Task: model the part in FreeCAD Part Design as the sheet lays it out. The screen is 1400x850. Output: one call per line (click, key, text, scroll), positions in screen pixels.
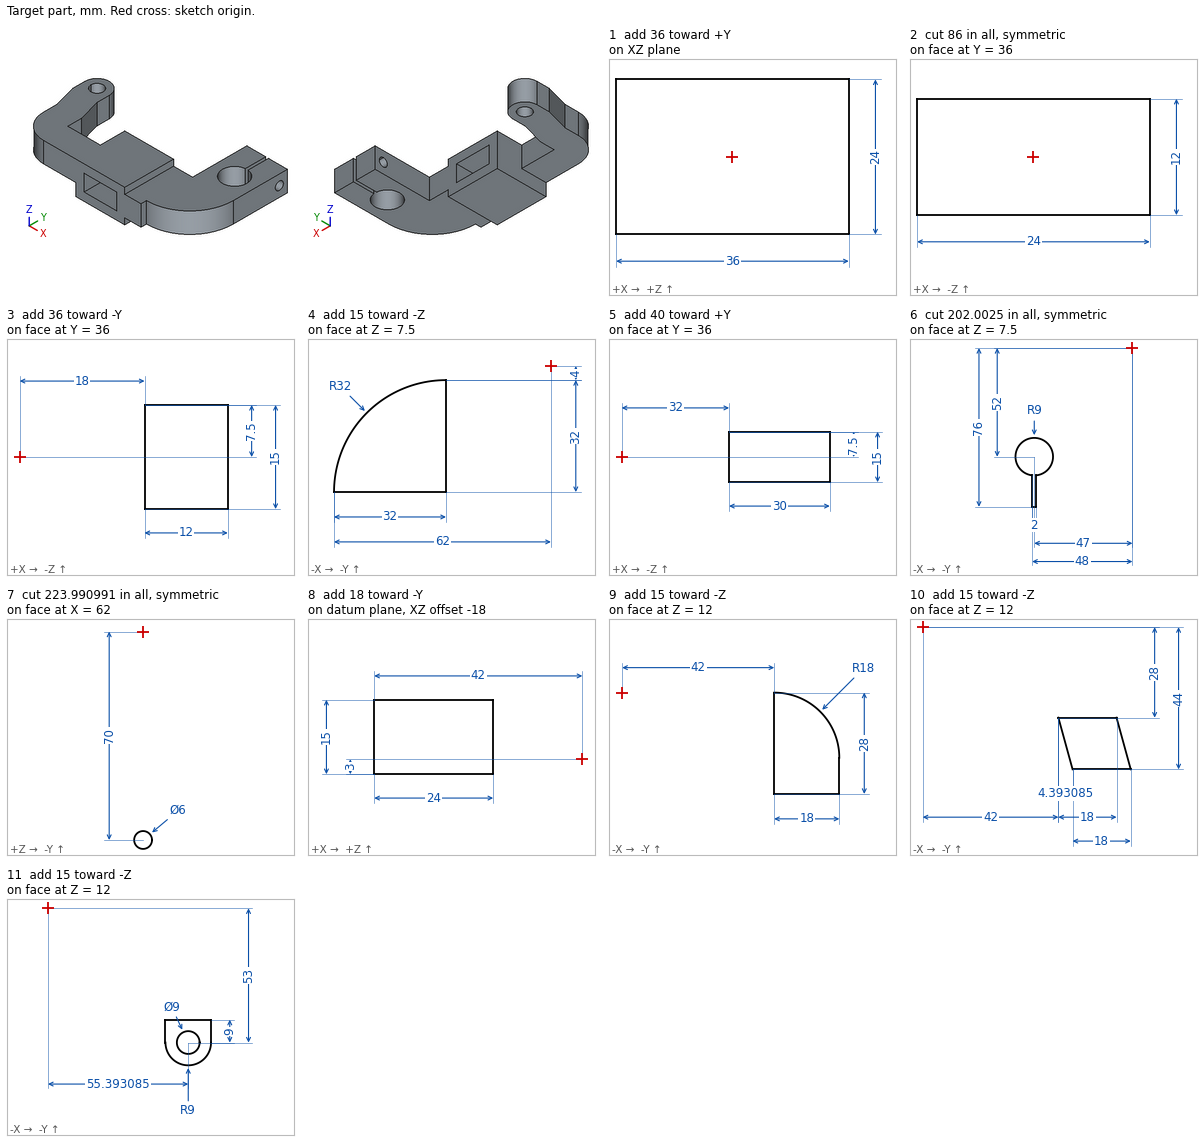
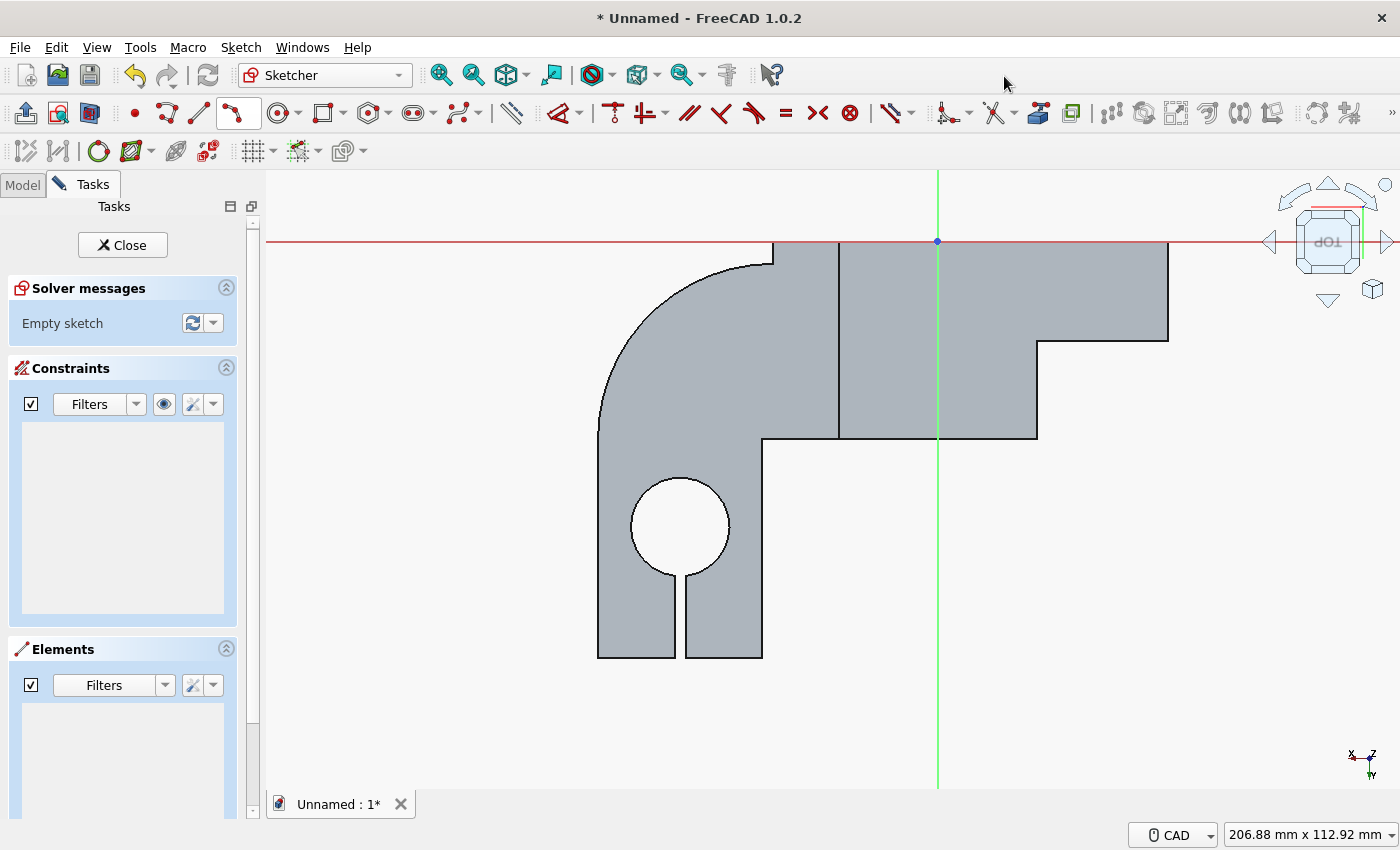
scroll(764, 480, down, 5)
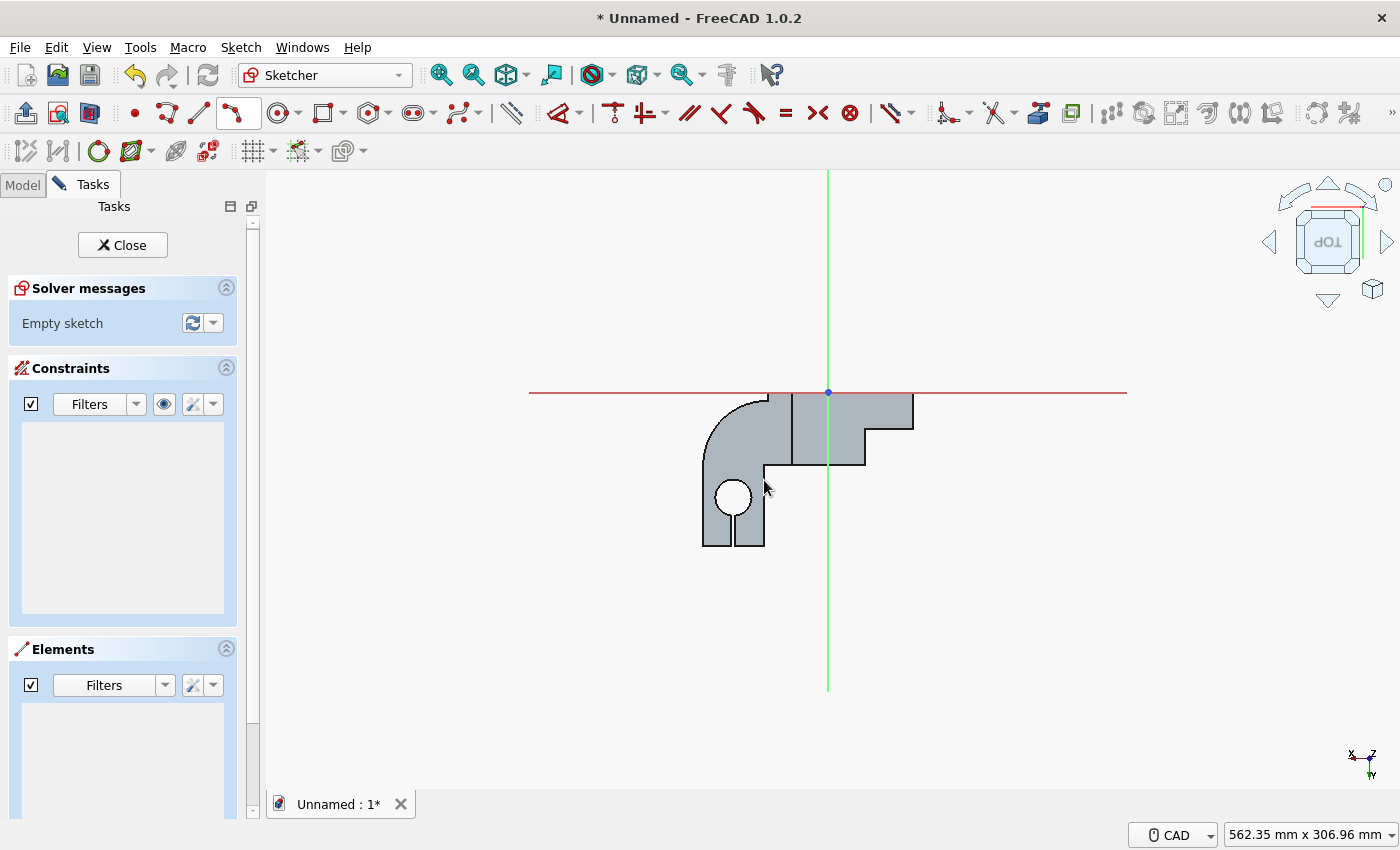
scroll(913, 409, up, 9)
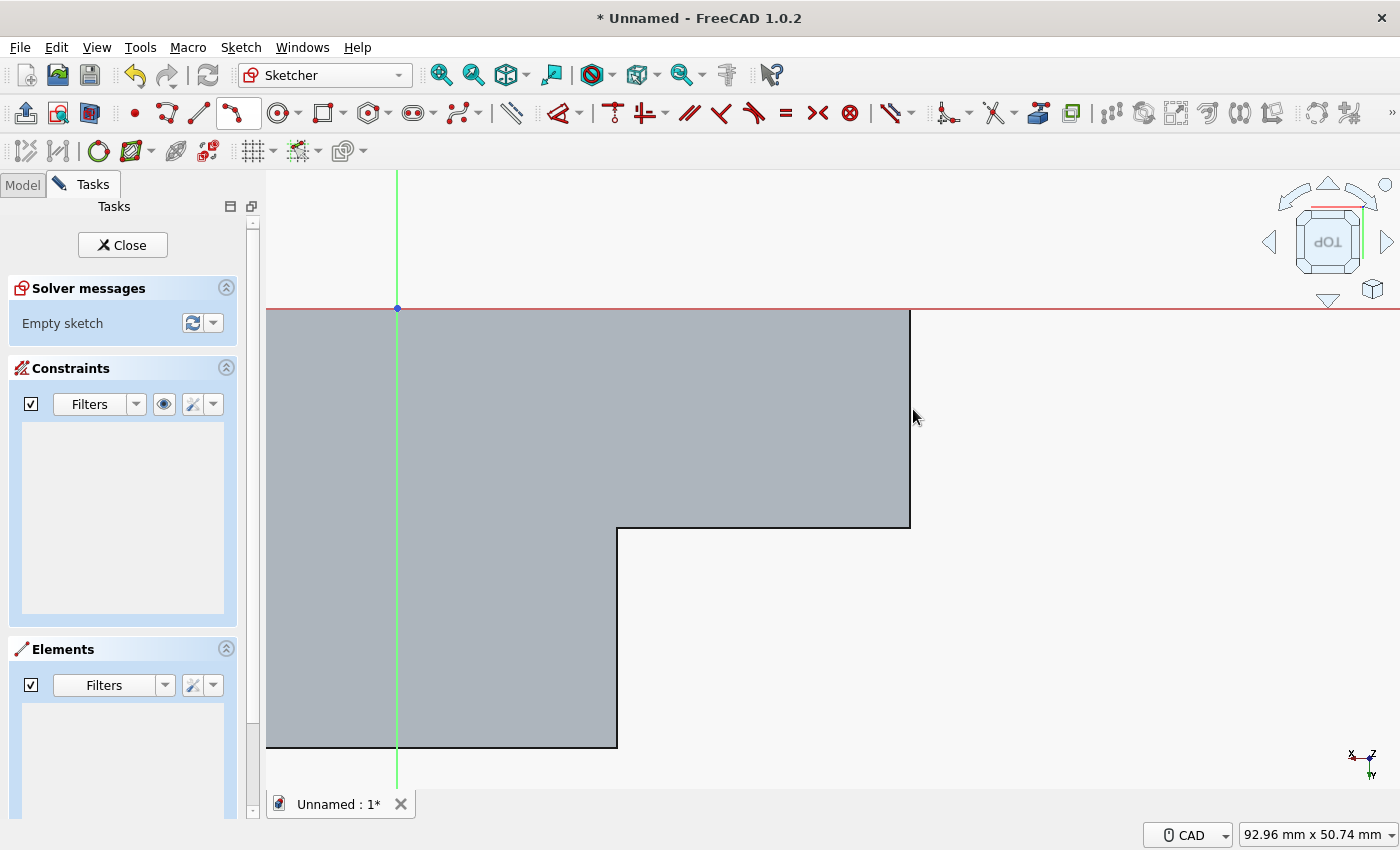
key(g)
key(m)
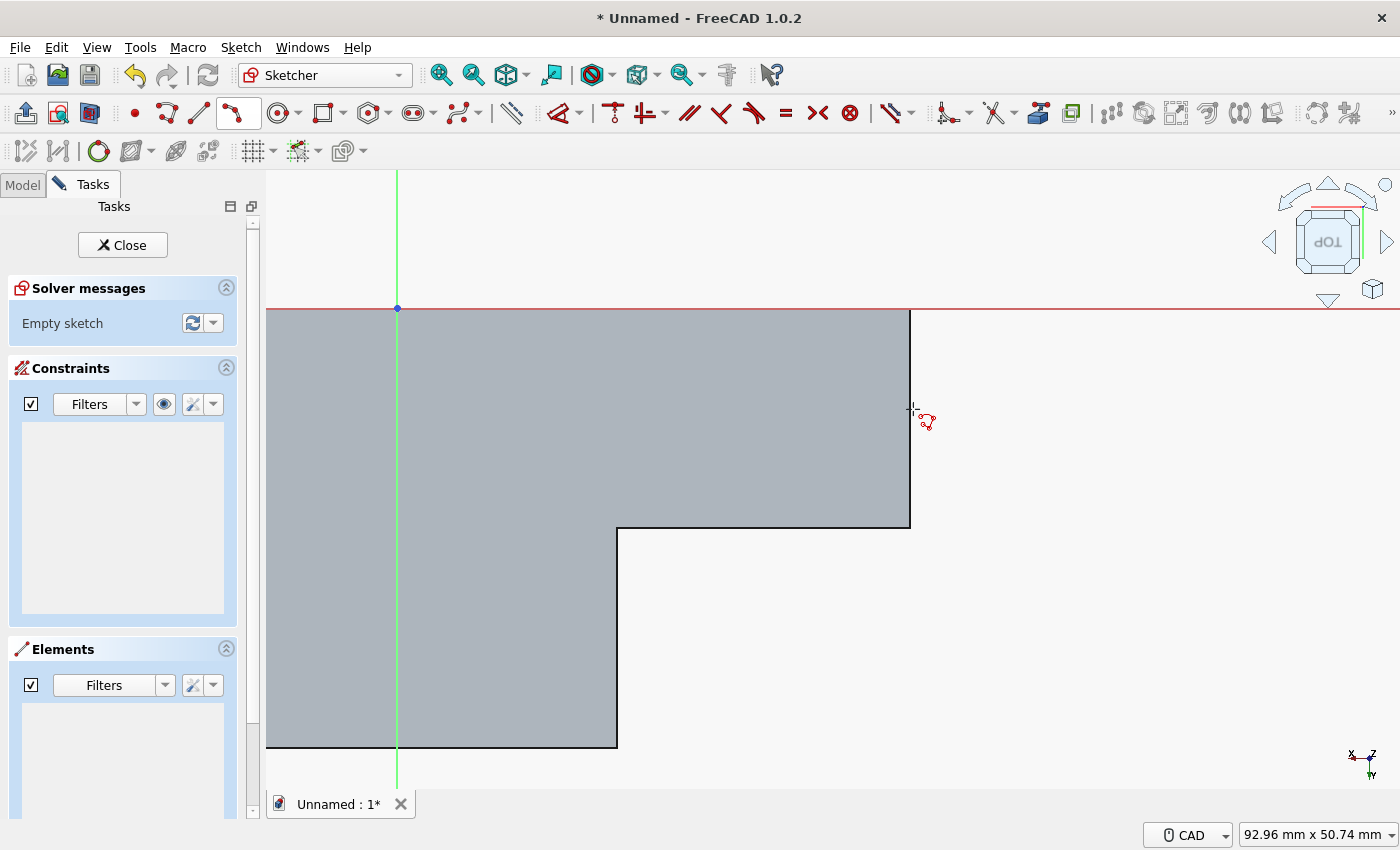
click(910, 309)
click(910, 650)
click(1129, 650)
click(1129, 528)
right_click(1129, 528)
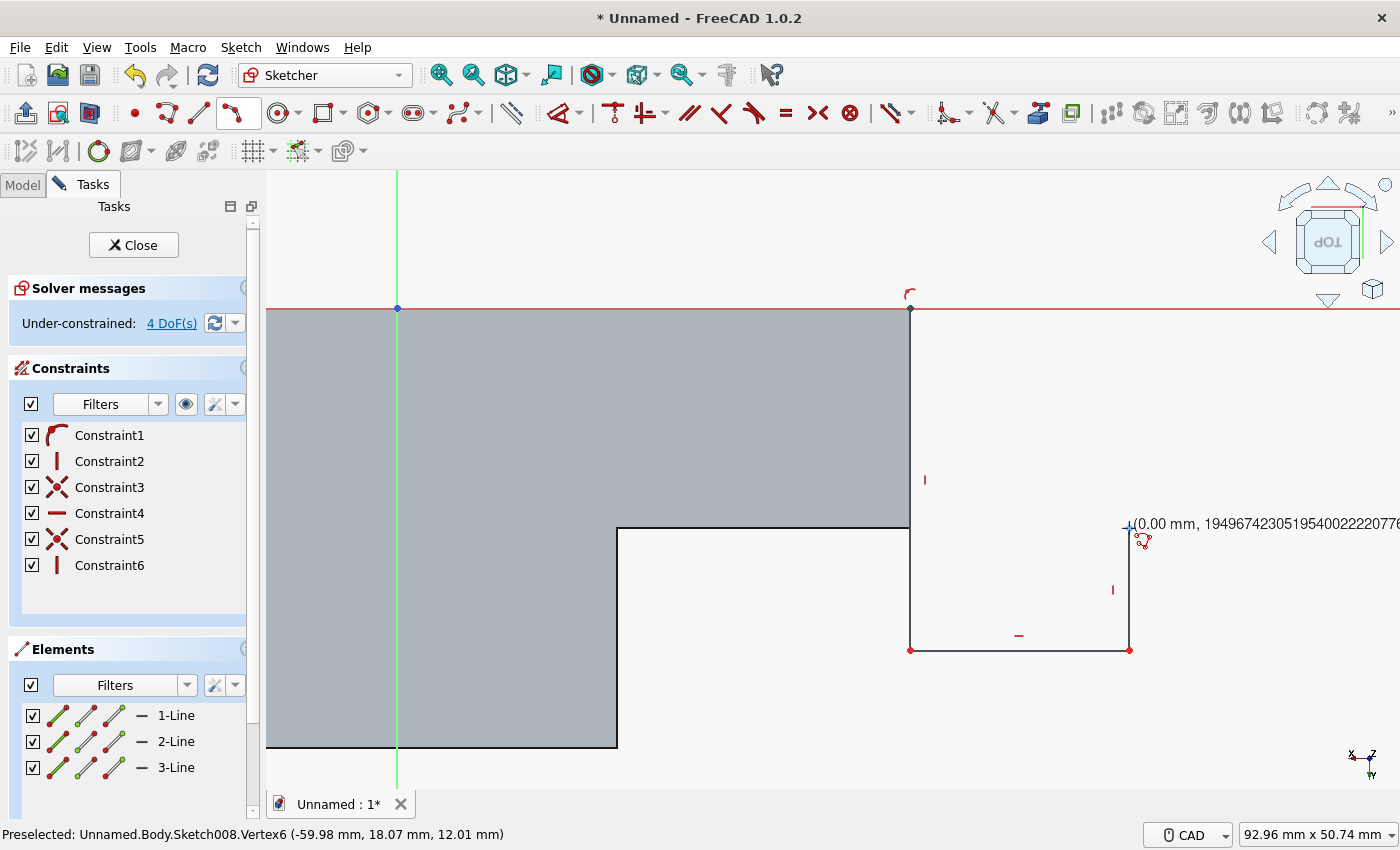
key(g)
key(3)
key(a)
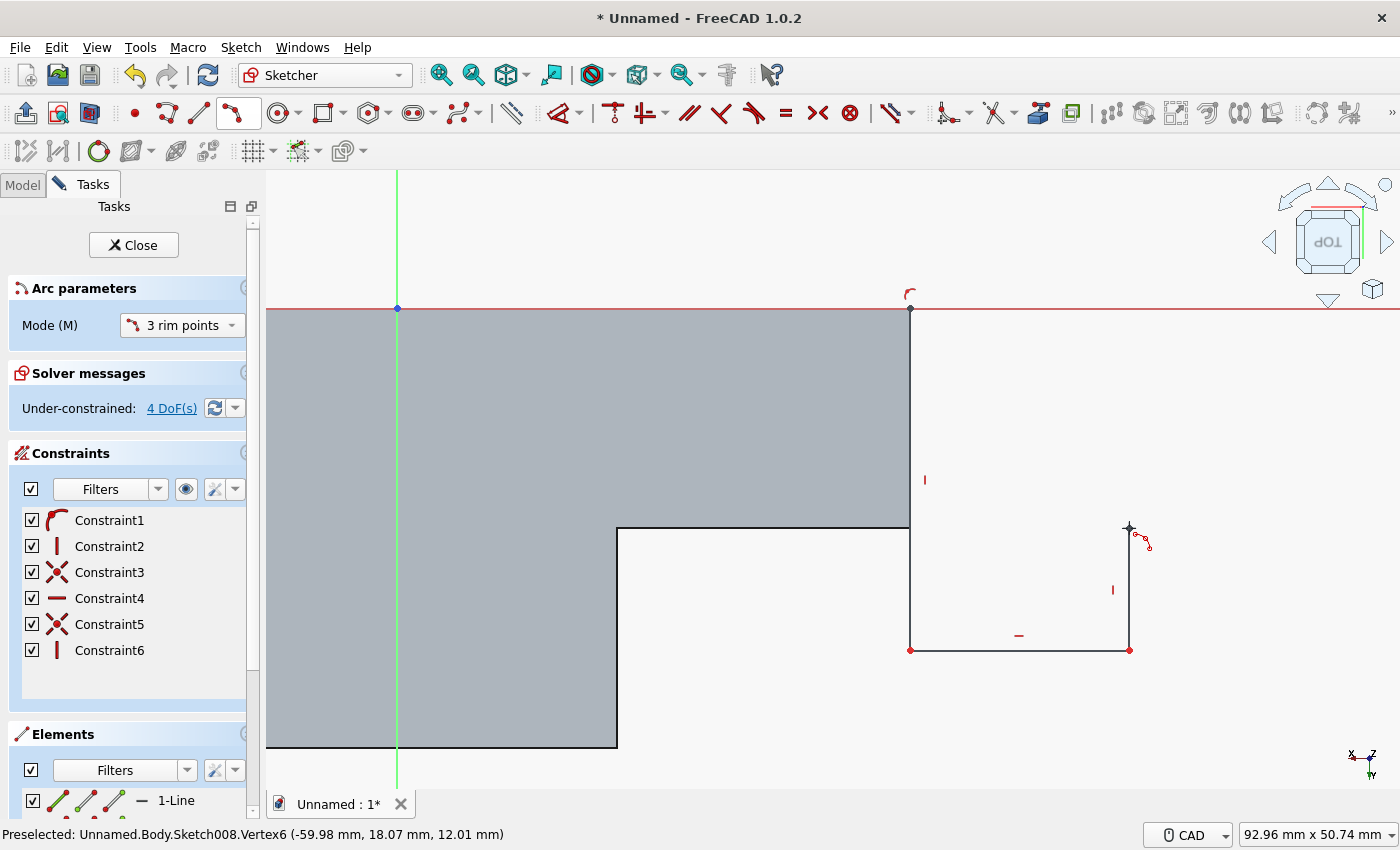
click(1129, 529)
click(910, 309)
click(1065, 373)
key(Escape)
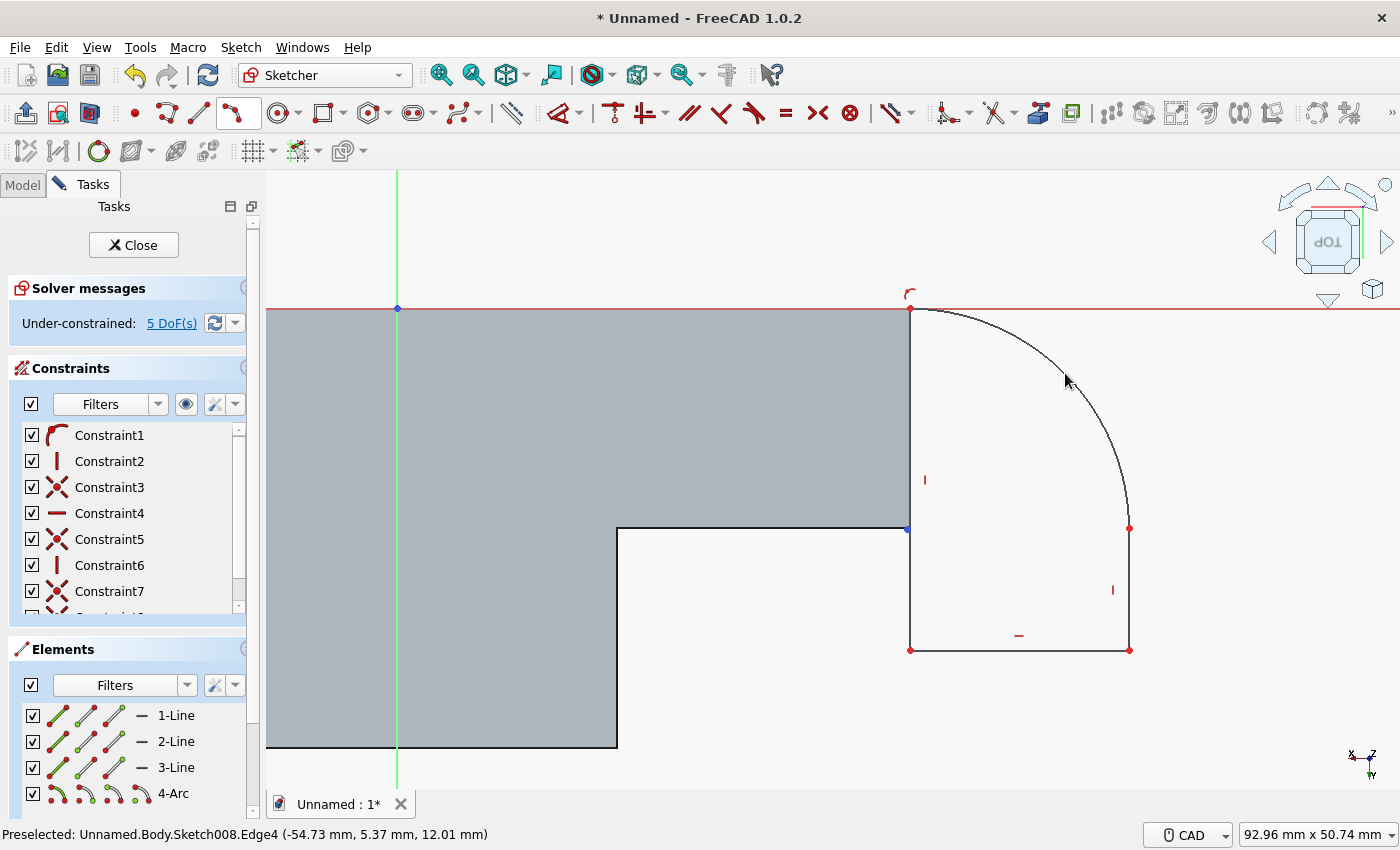
click(1129, 614)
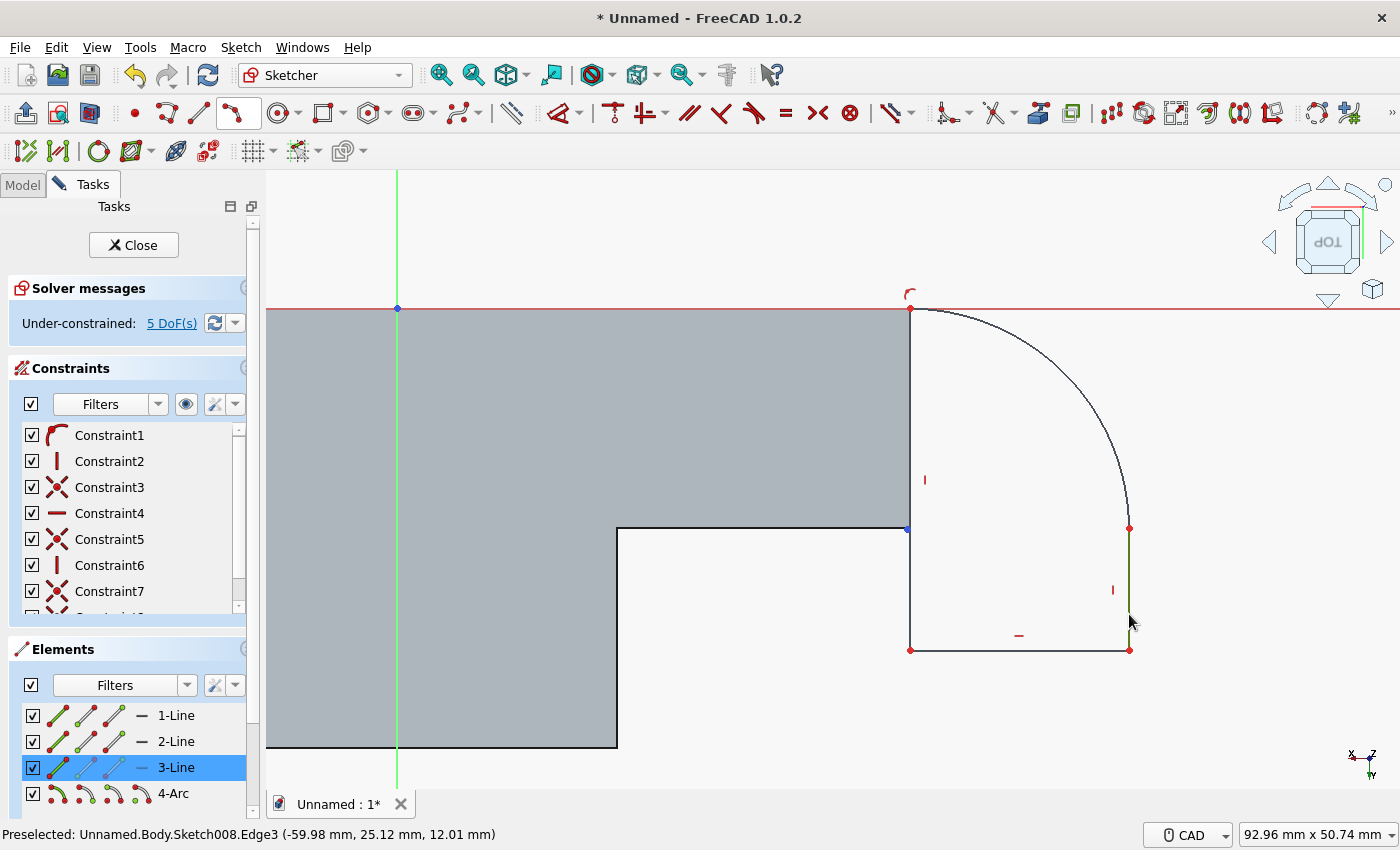
click(1105, 429)